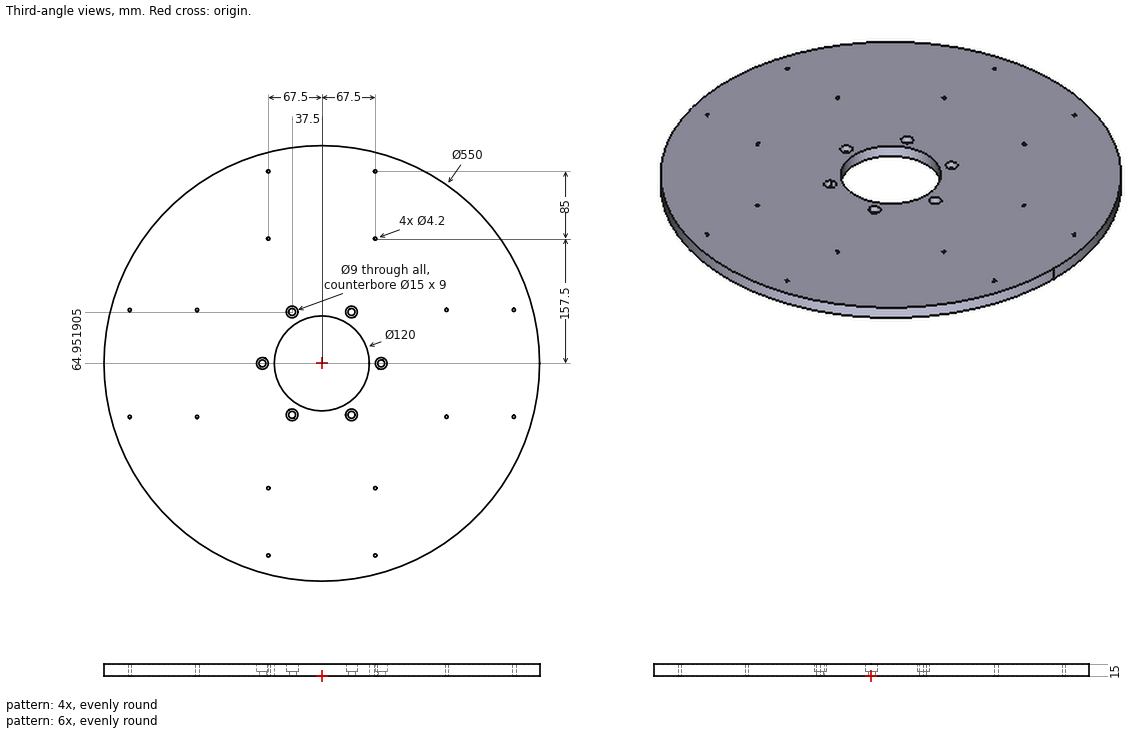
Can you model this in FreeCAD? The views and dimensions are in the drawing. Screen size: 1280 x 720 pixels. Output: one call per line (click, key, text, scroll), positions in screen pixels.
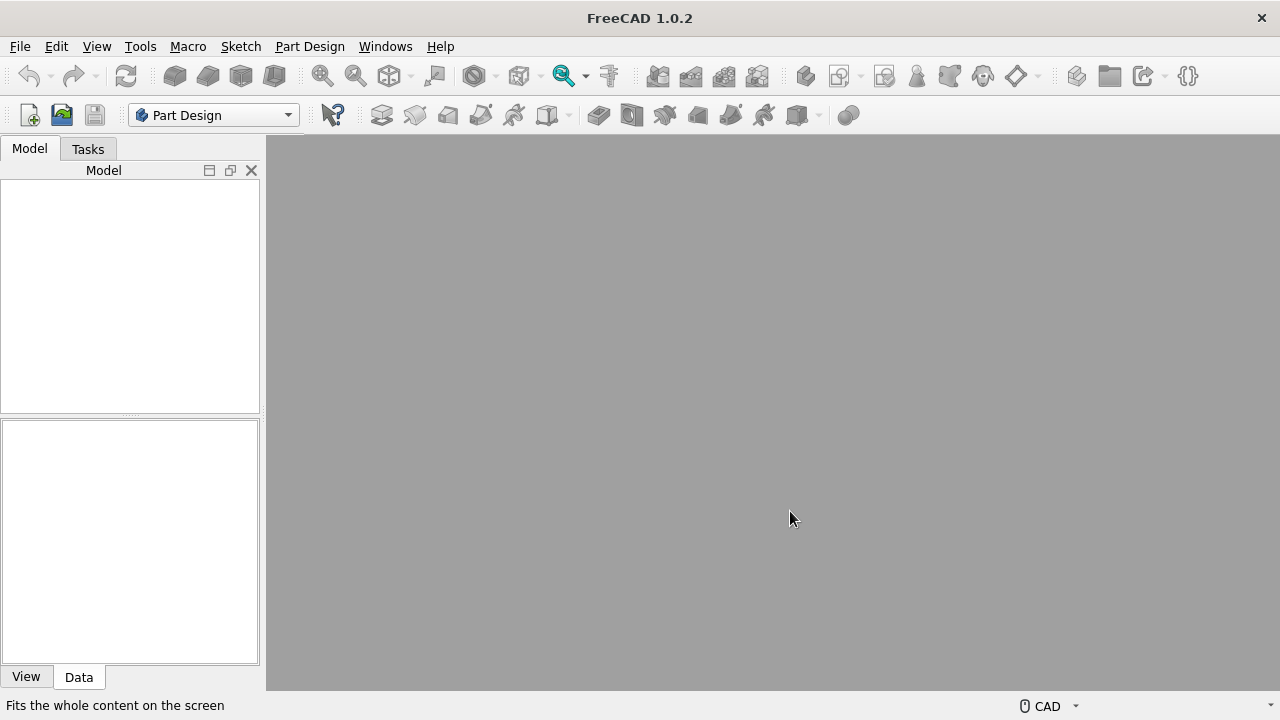
click(29, 116)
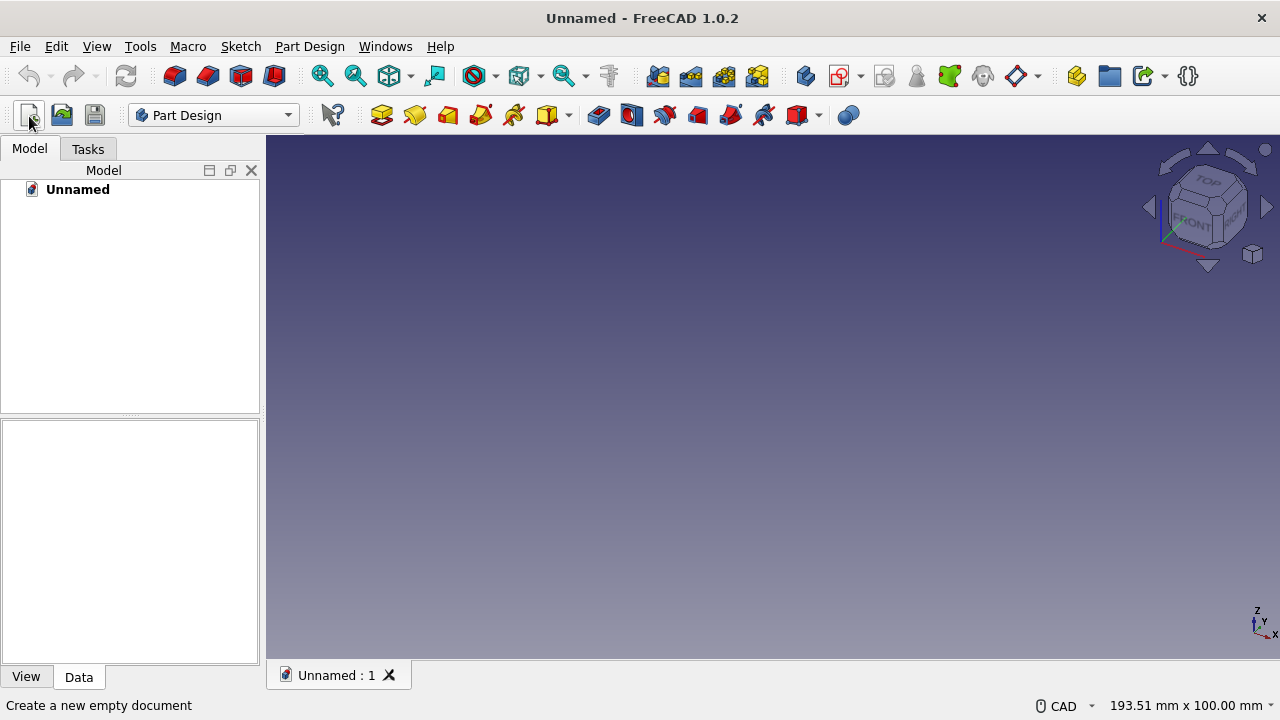
click(838, 76)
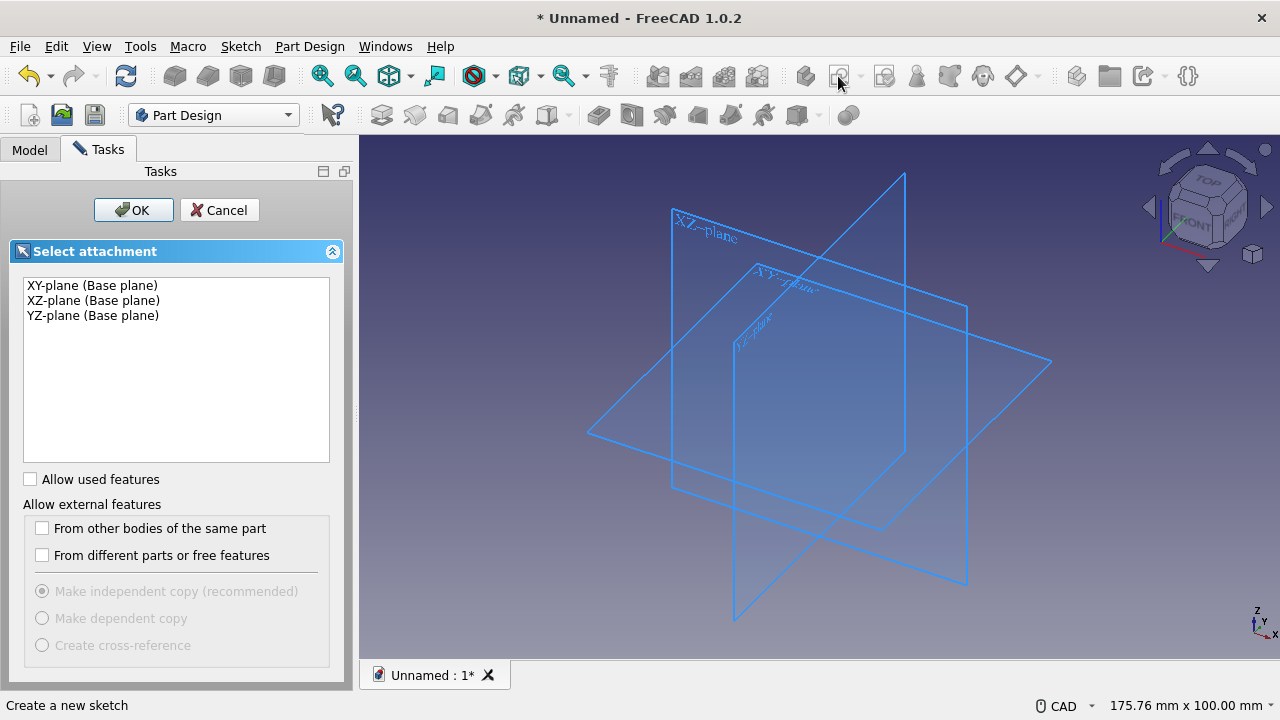
click(84, 286)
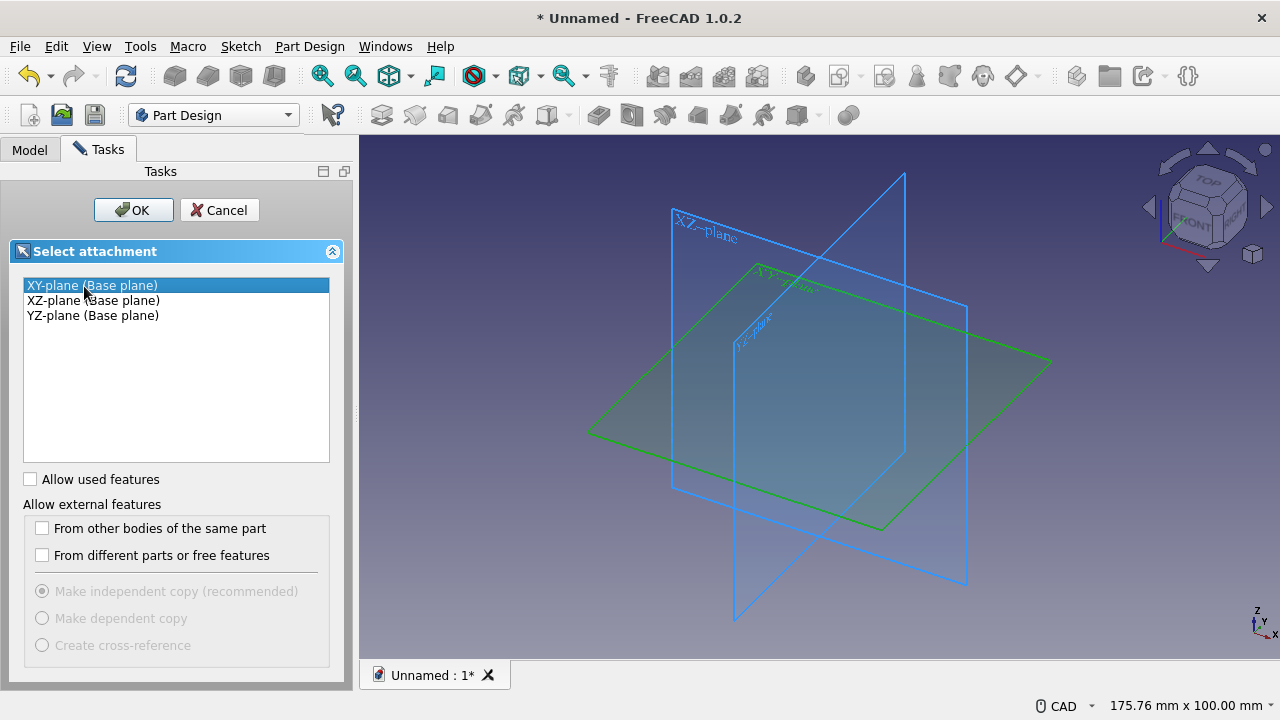
click(134, 210)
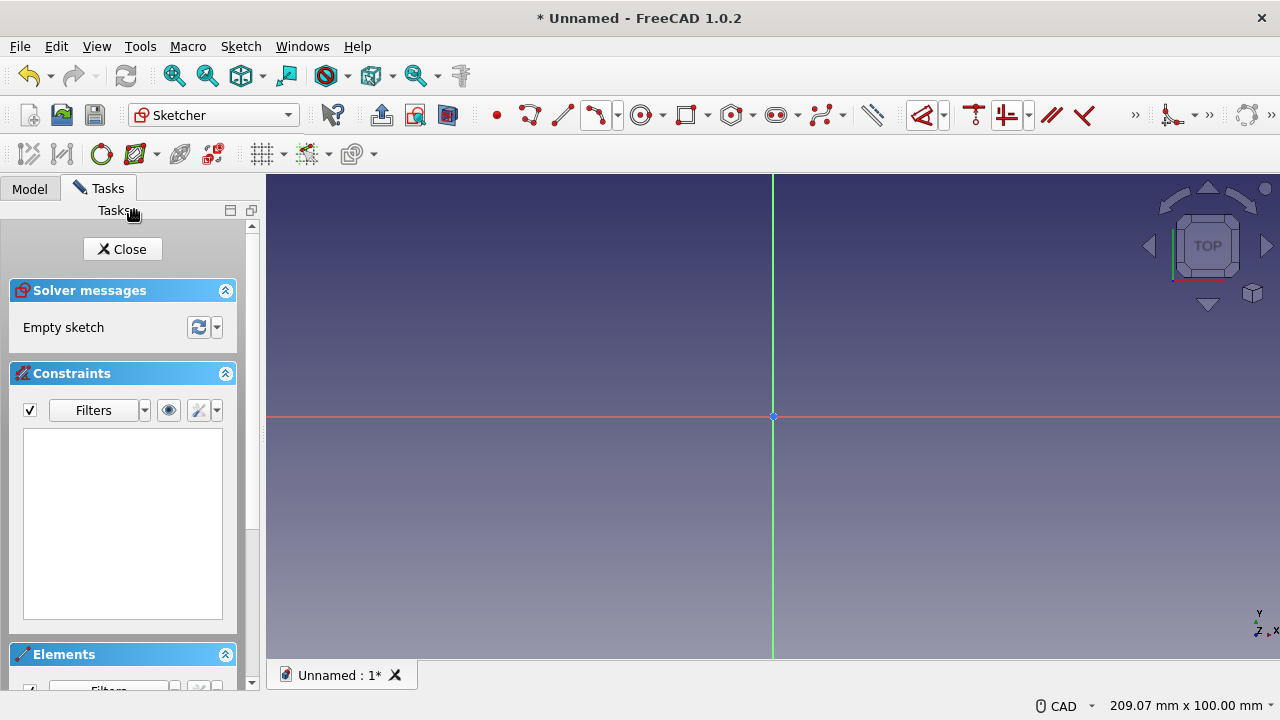
scroll(696, 416, down, 11)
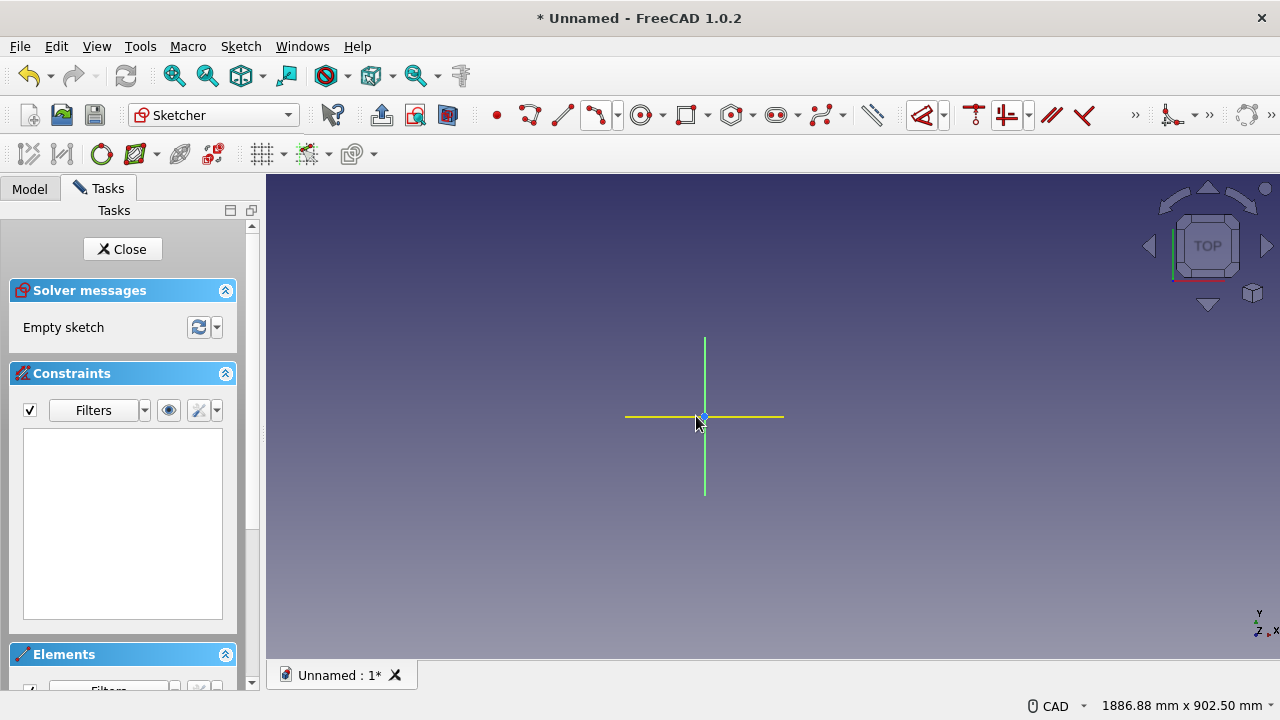
click(640, 116)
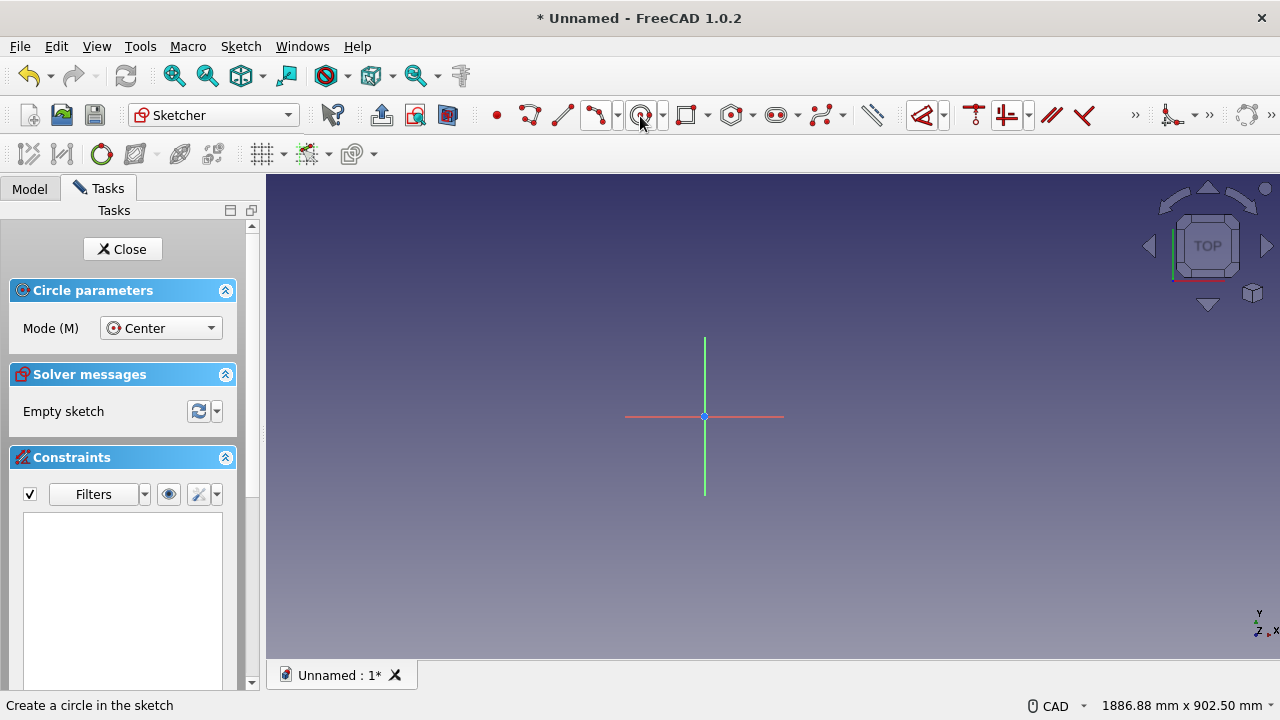
click(705, 416)
move(809, 312)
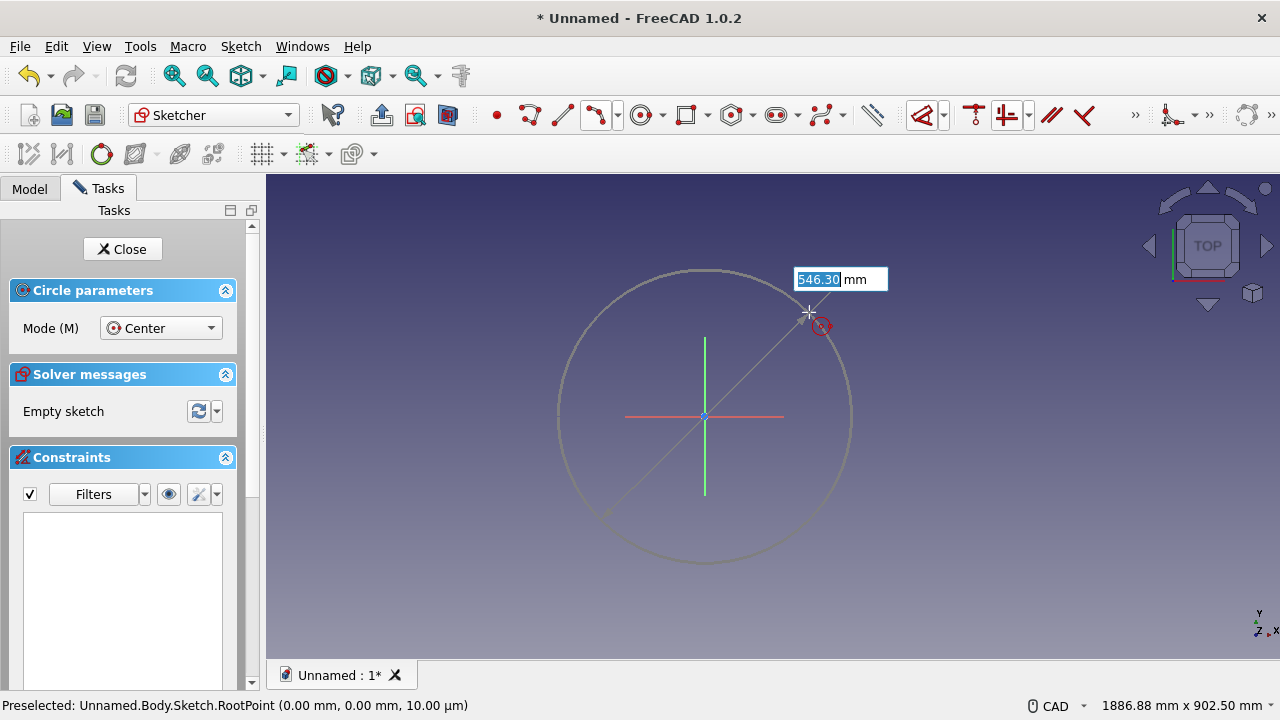
text(550)
key(Return)
key(Escape)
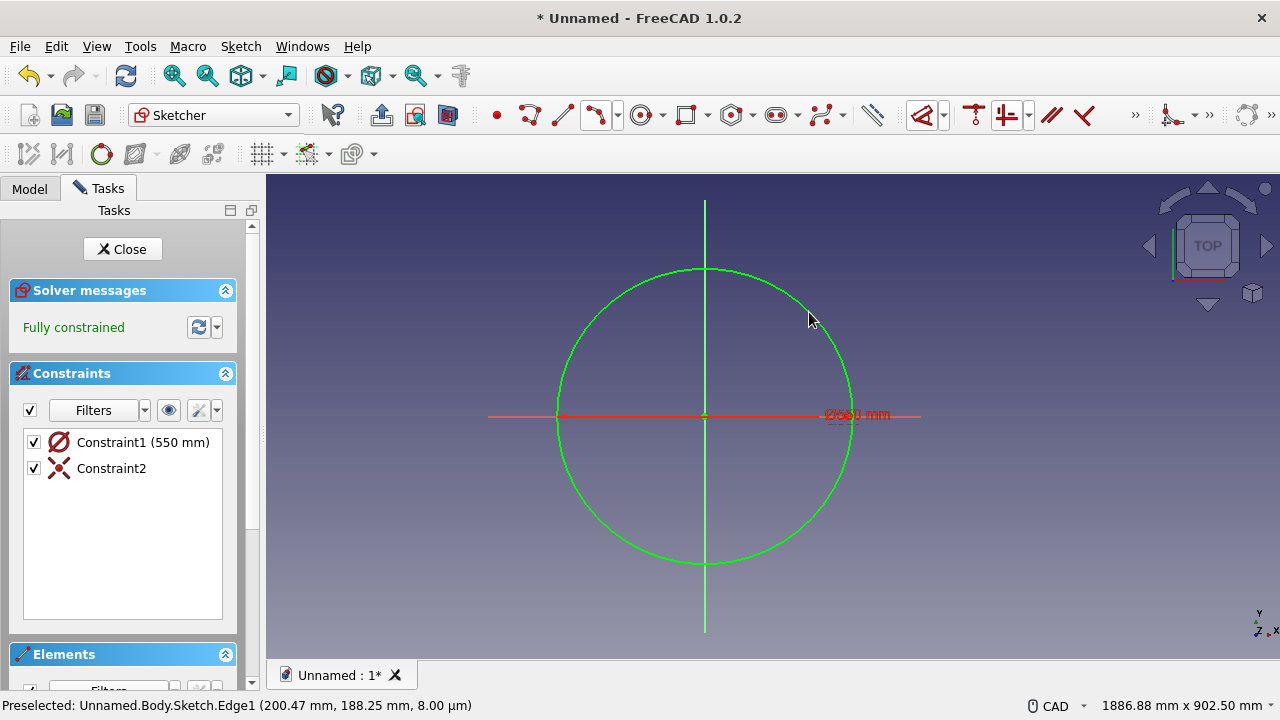
click(123, 249)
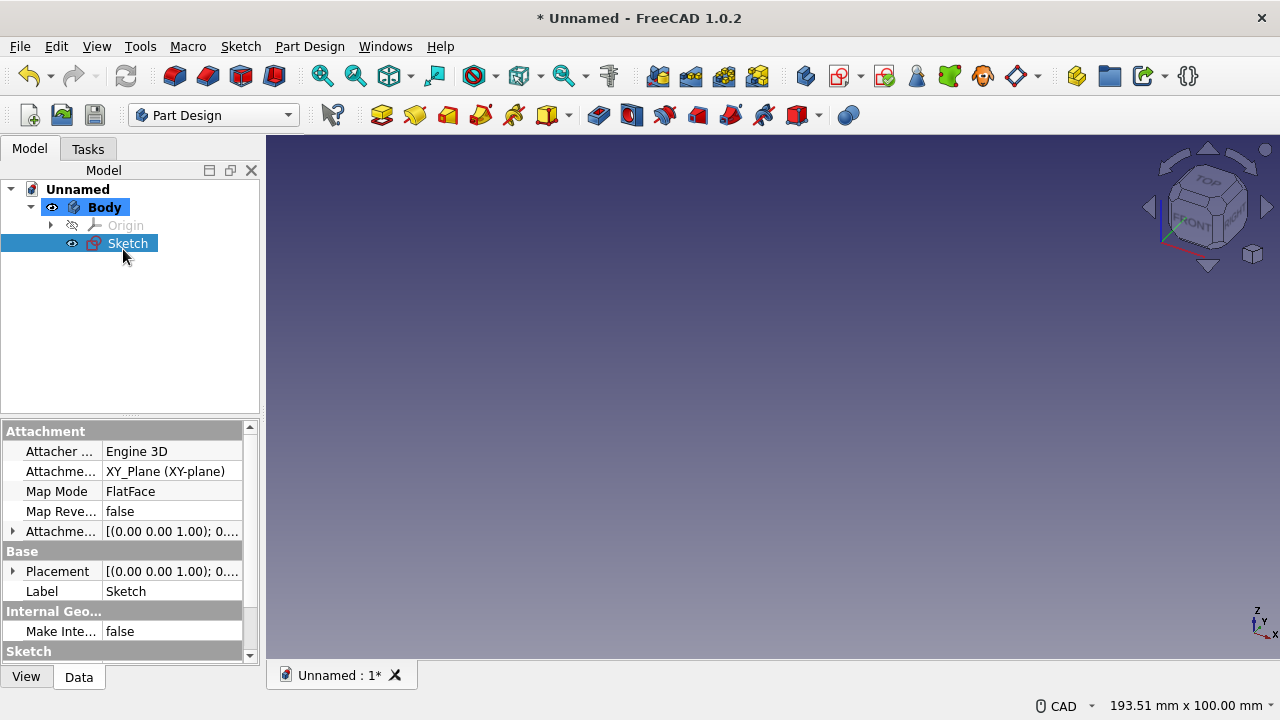
click(382, 116)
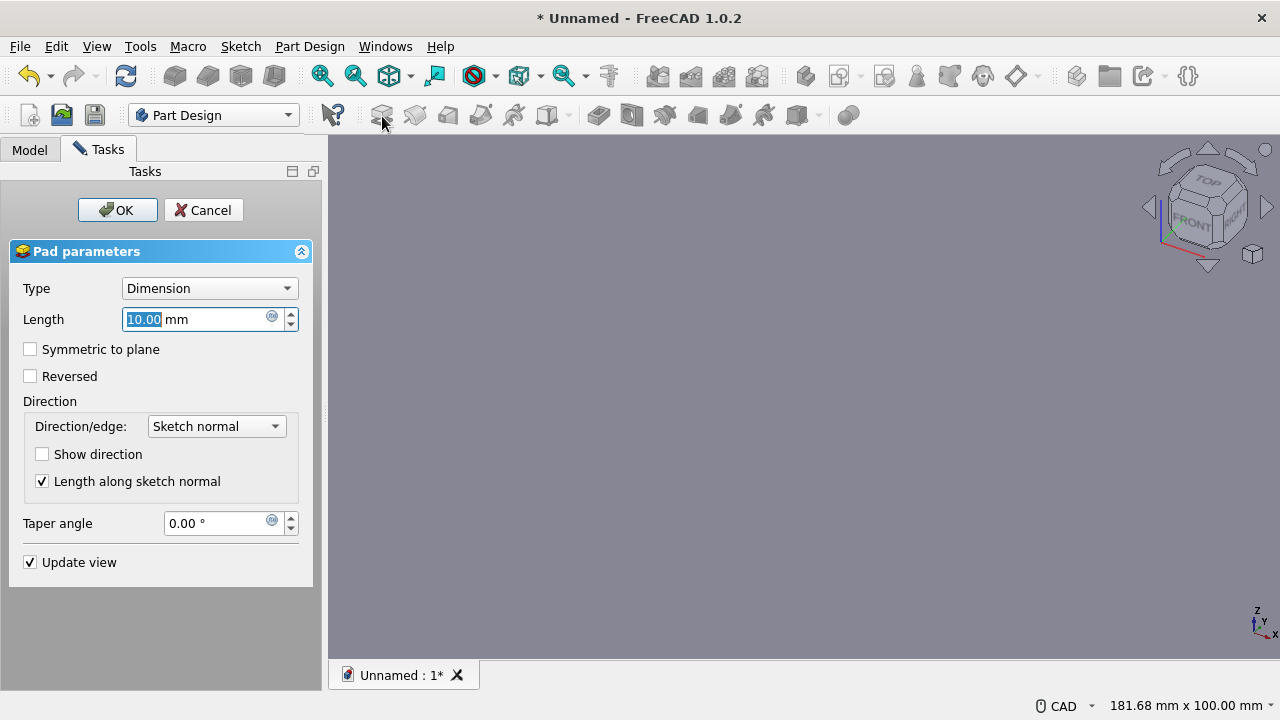
text(15)
key(Tab)